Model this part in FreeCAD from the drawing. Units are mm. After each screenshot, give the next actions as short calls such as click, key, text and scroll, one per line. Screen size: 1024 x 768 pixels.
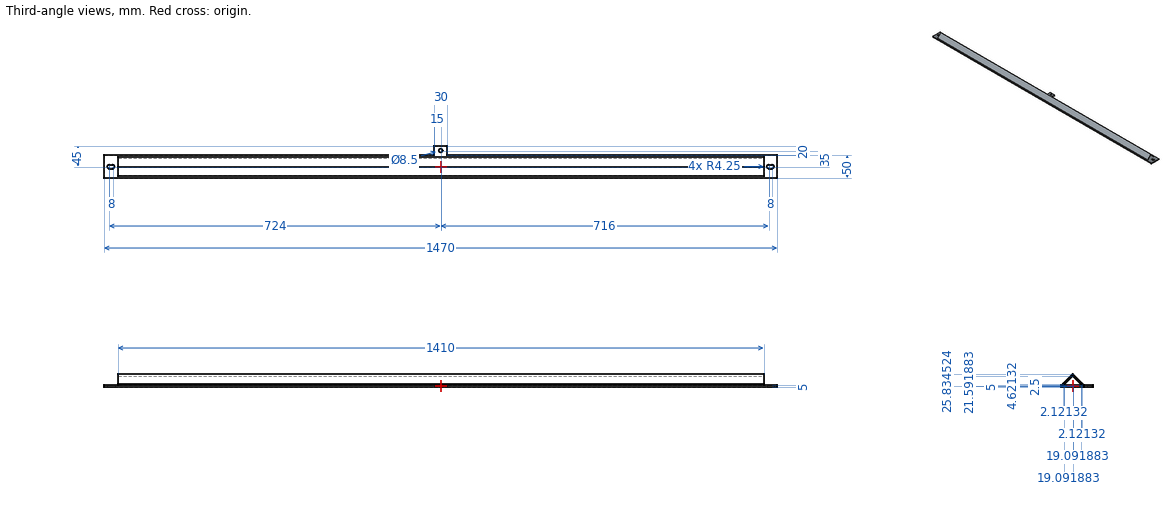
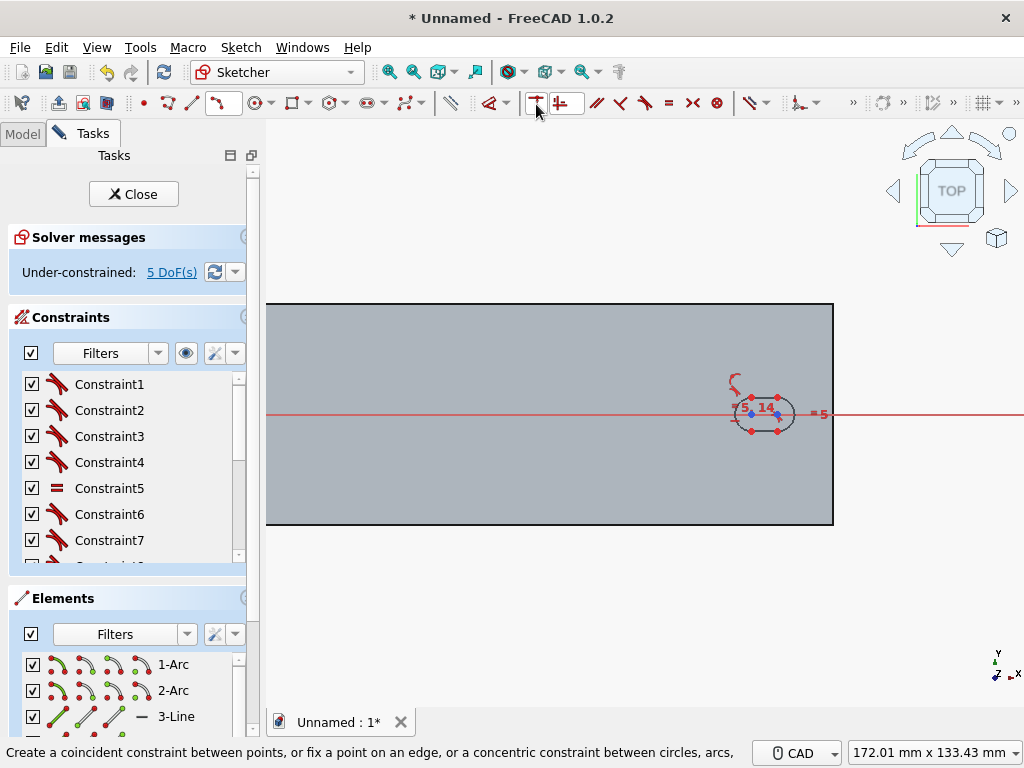
scroll(738, 405, up, 4)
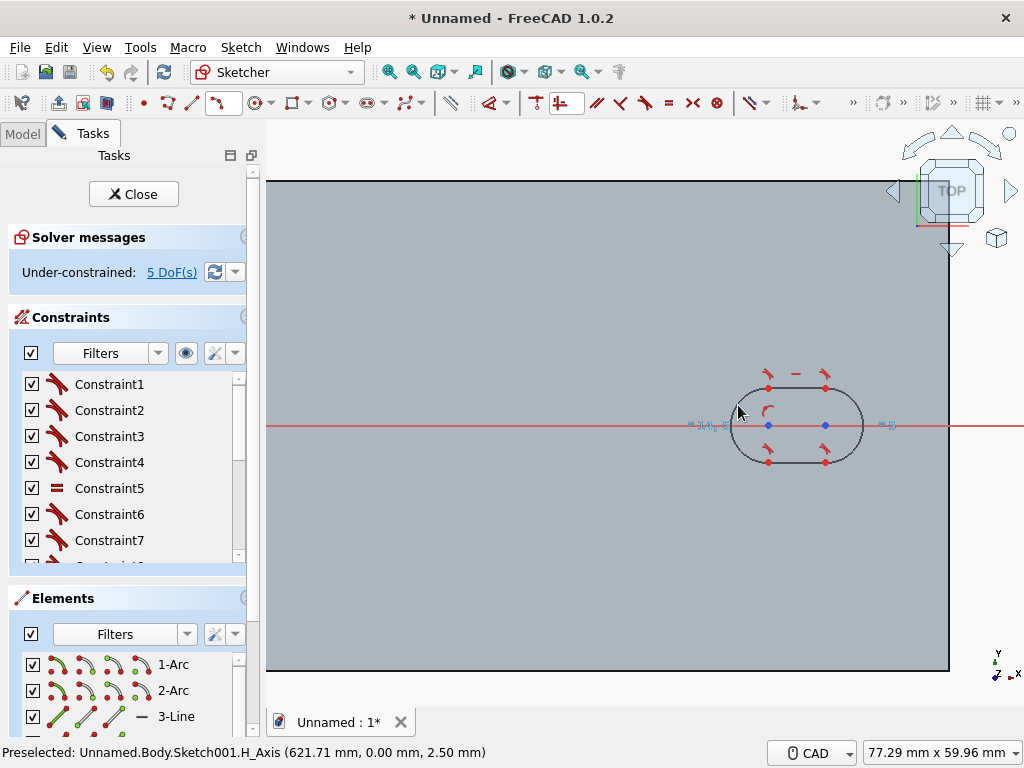
click(738, 404)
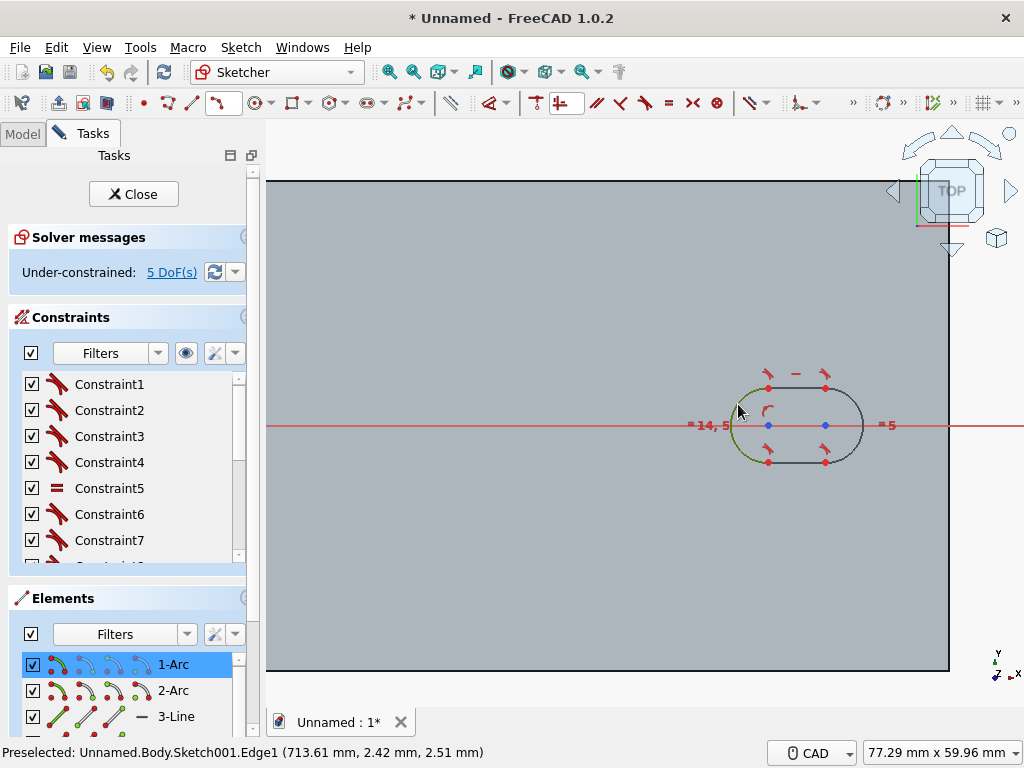
click(508, 104)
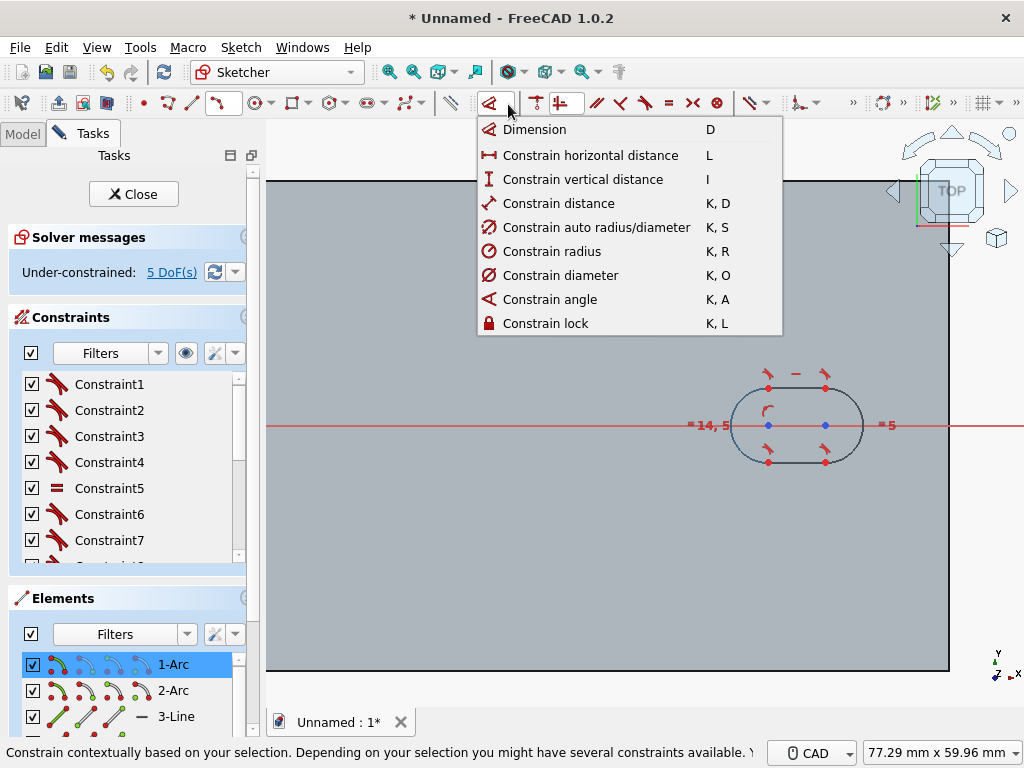
click(630, 251)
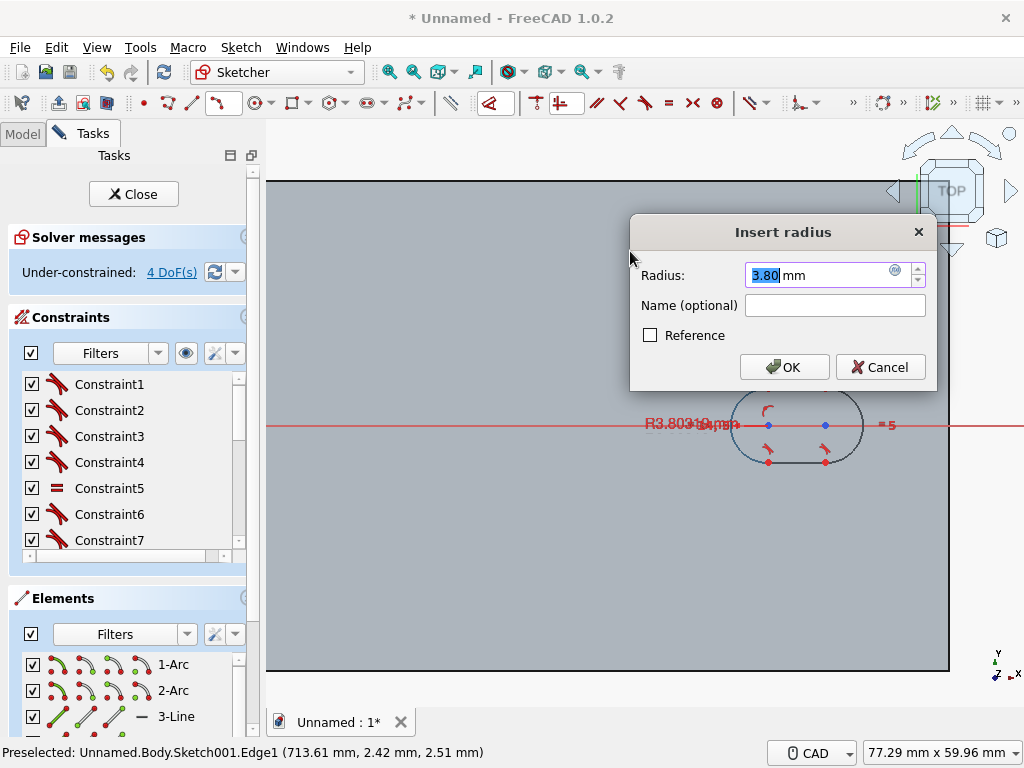
text(4.25)
key(Return)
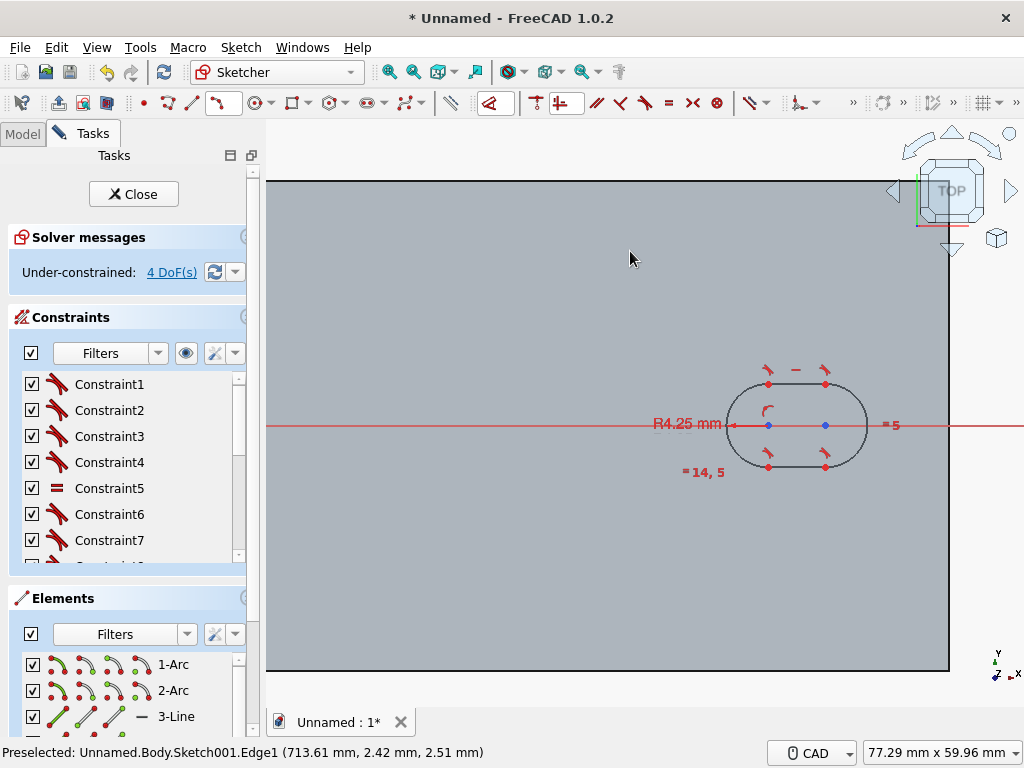
click(785, 384)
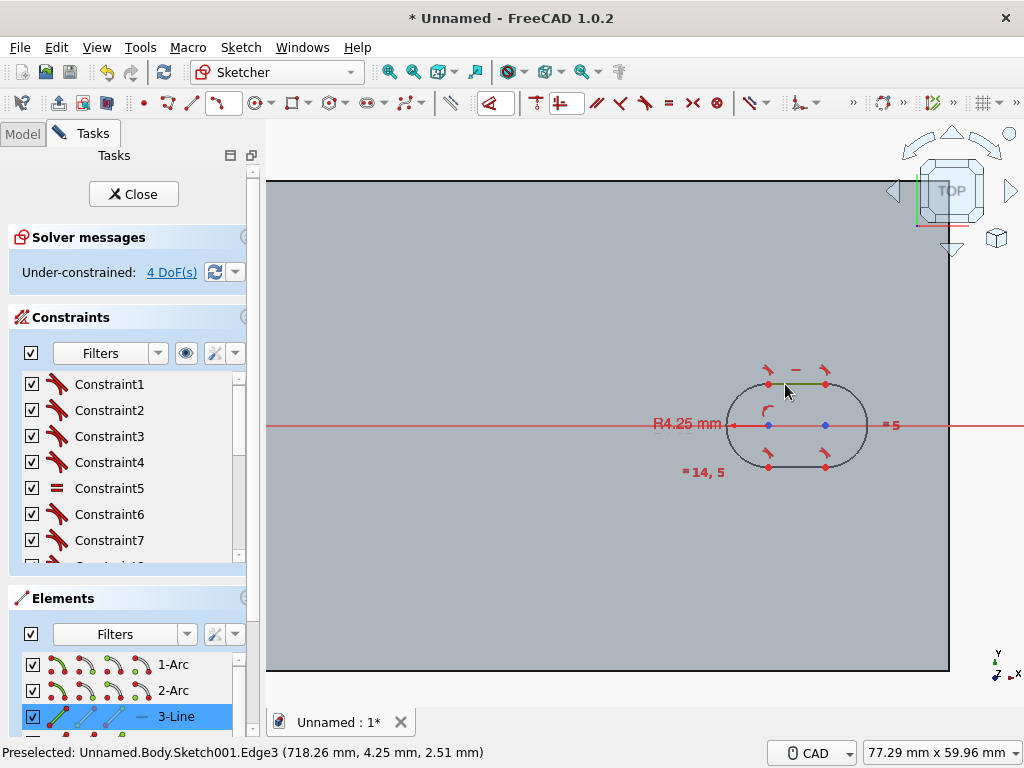
click(508, 104)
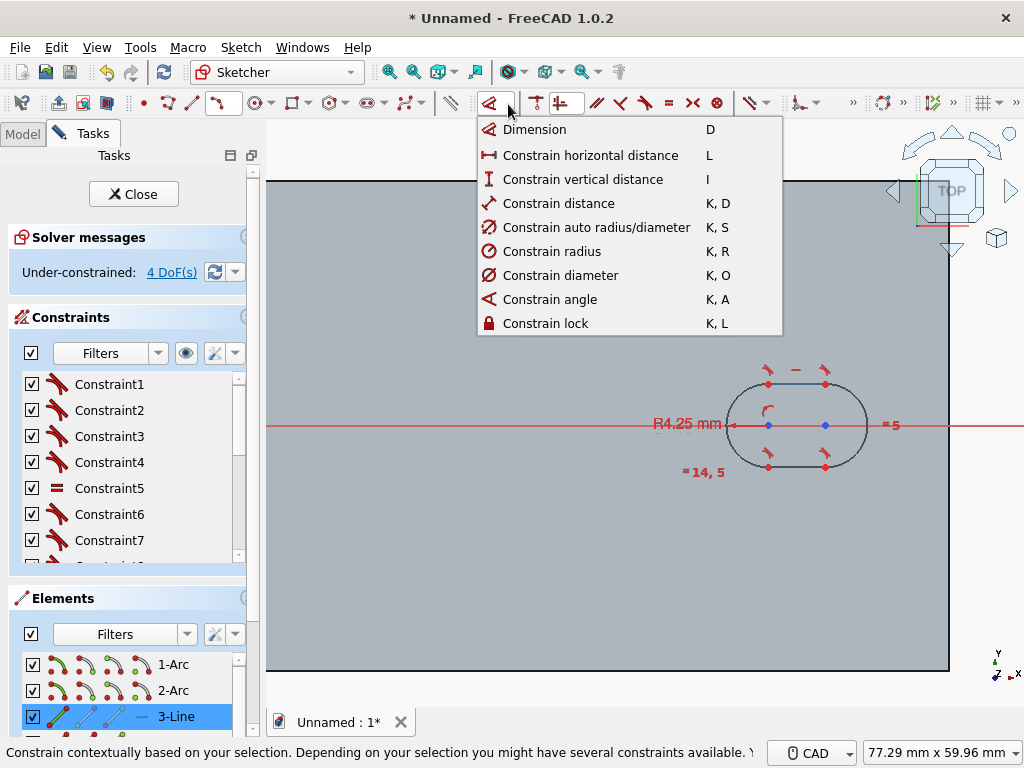
click(630, 155)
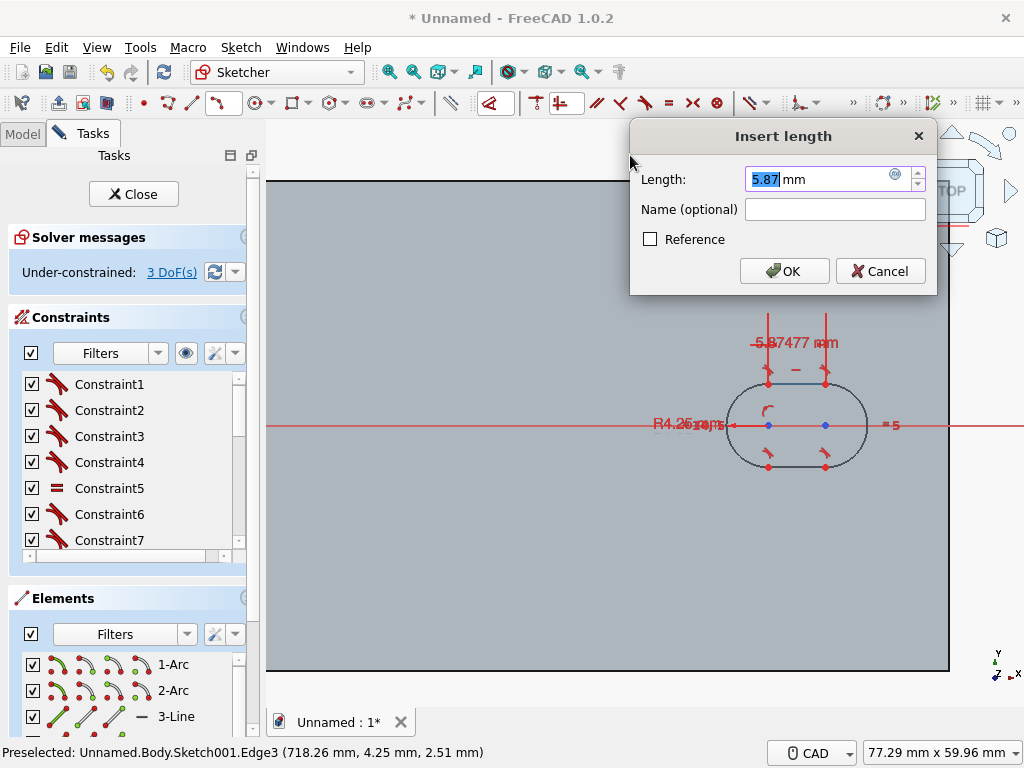
text(8)
key(Return)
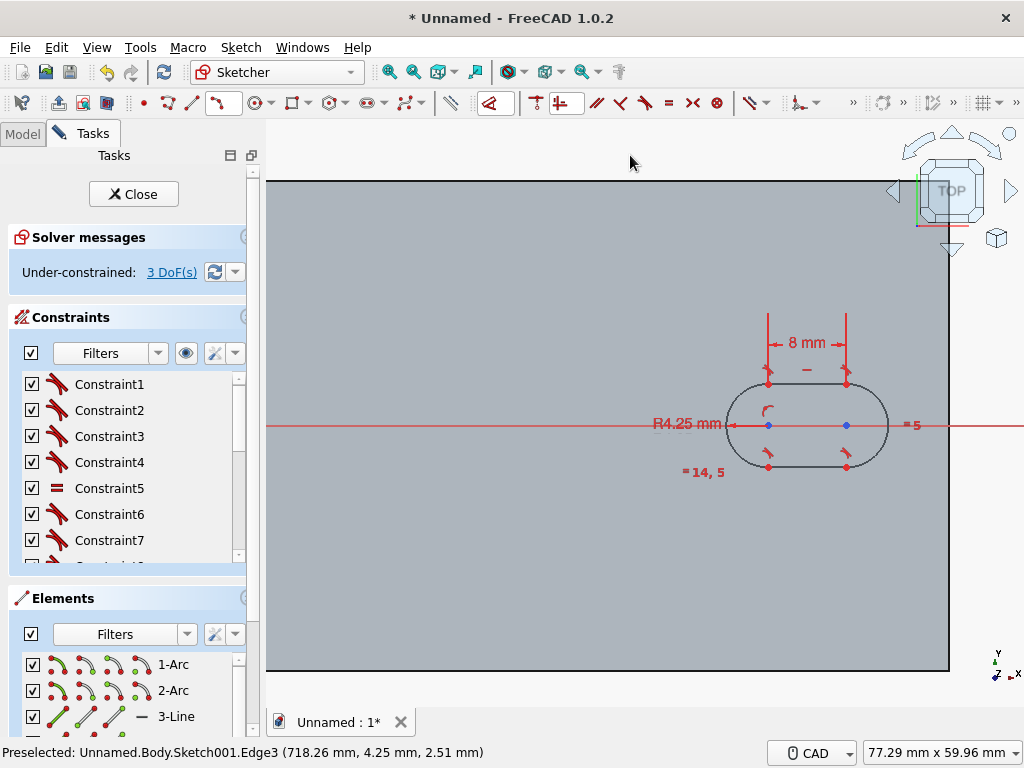
scroll(813, 413, down, 17)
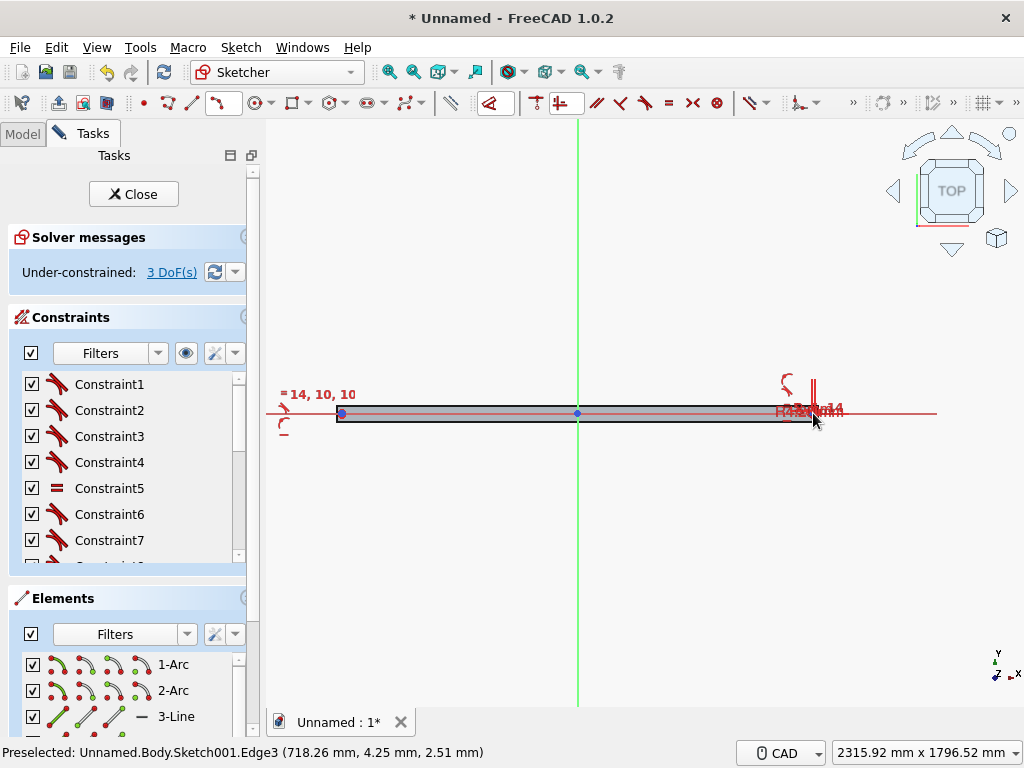
scroll(342, 413, up, 14)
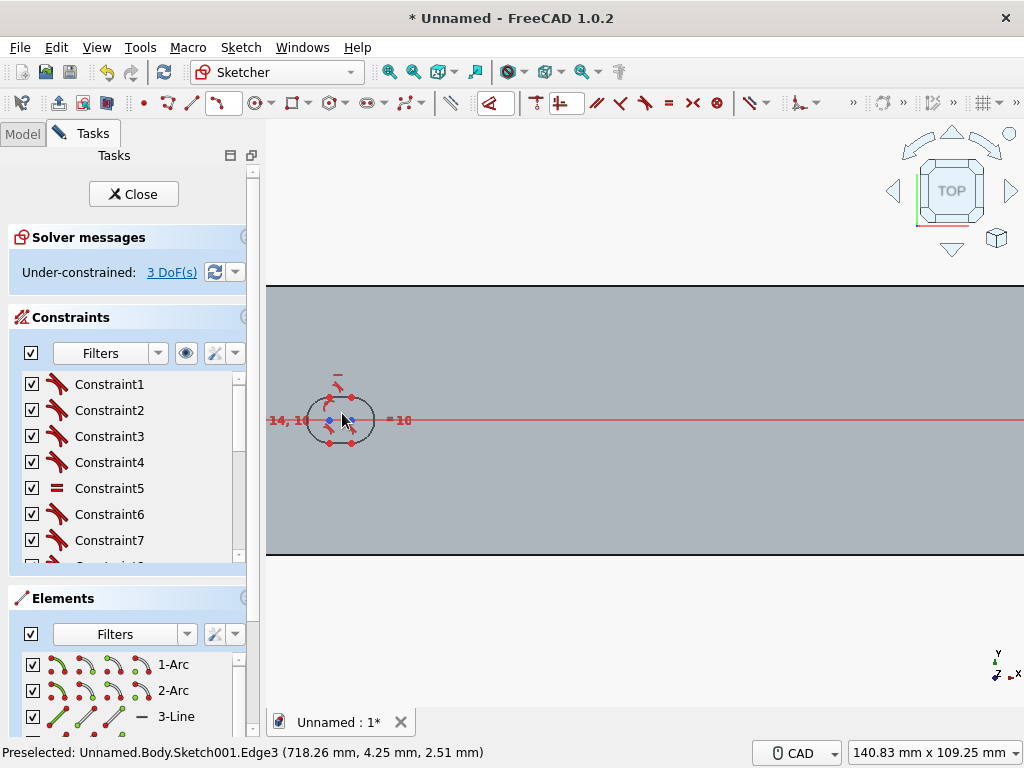
click(336, 397)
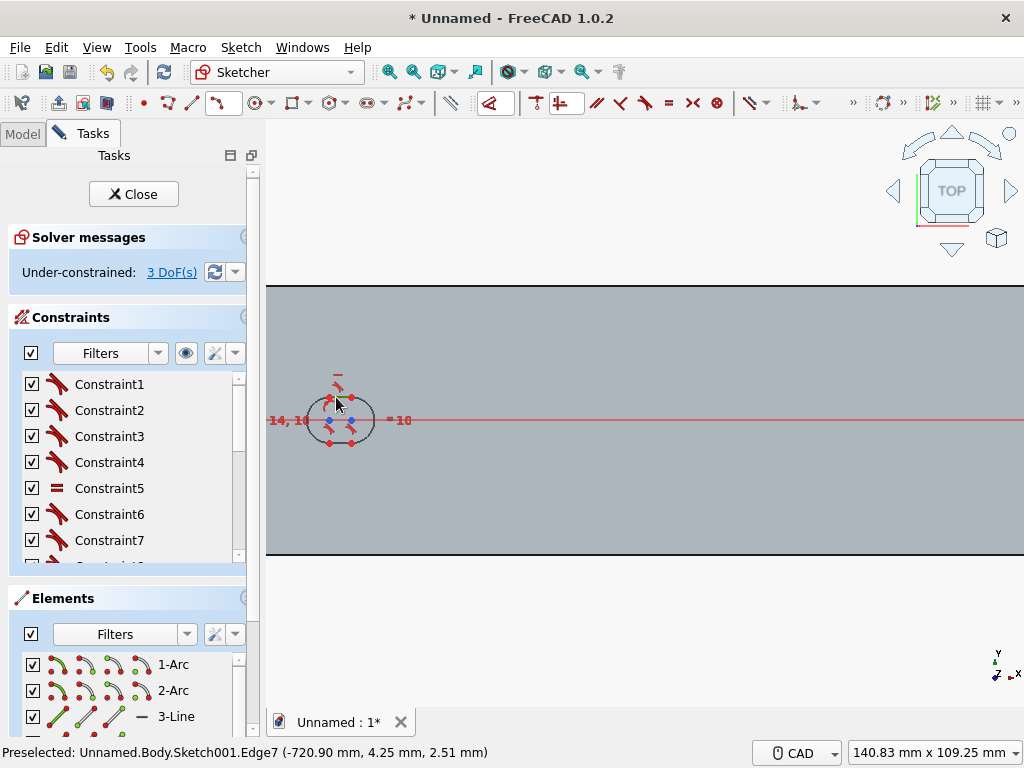
click(508, 104)